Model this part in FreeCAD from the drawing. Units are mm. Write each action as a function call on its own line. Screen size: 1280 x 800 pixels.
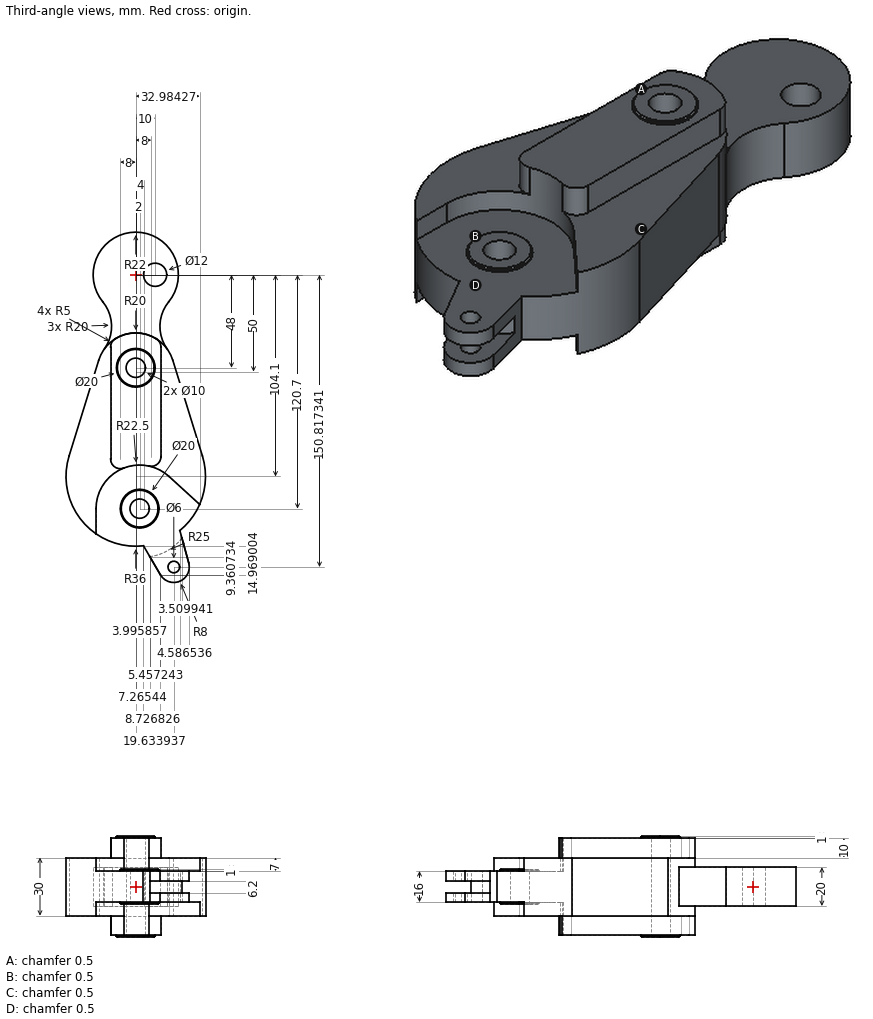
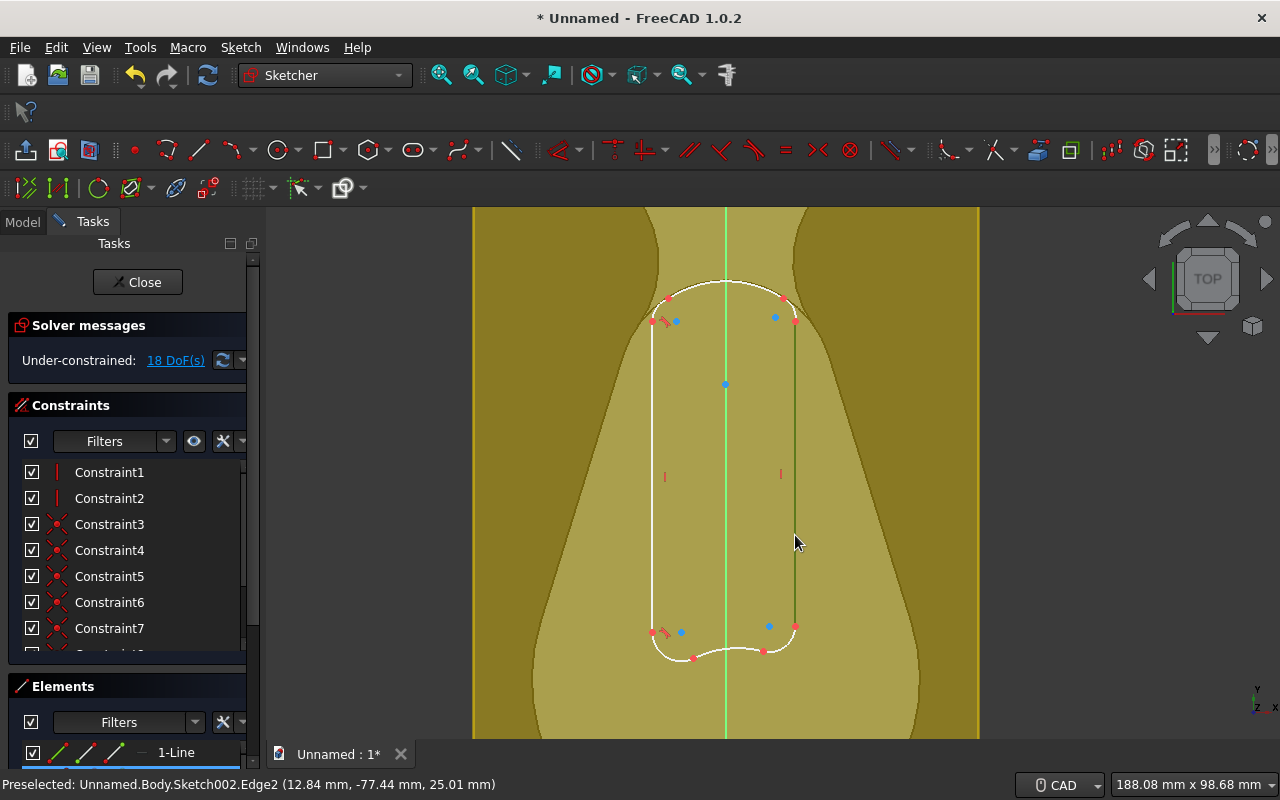
click(777, 651)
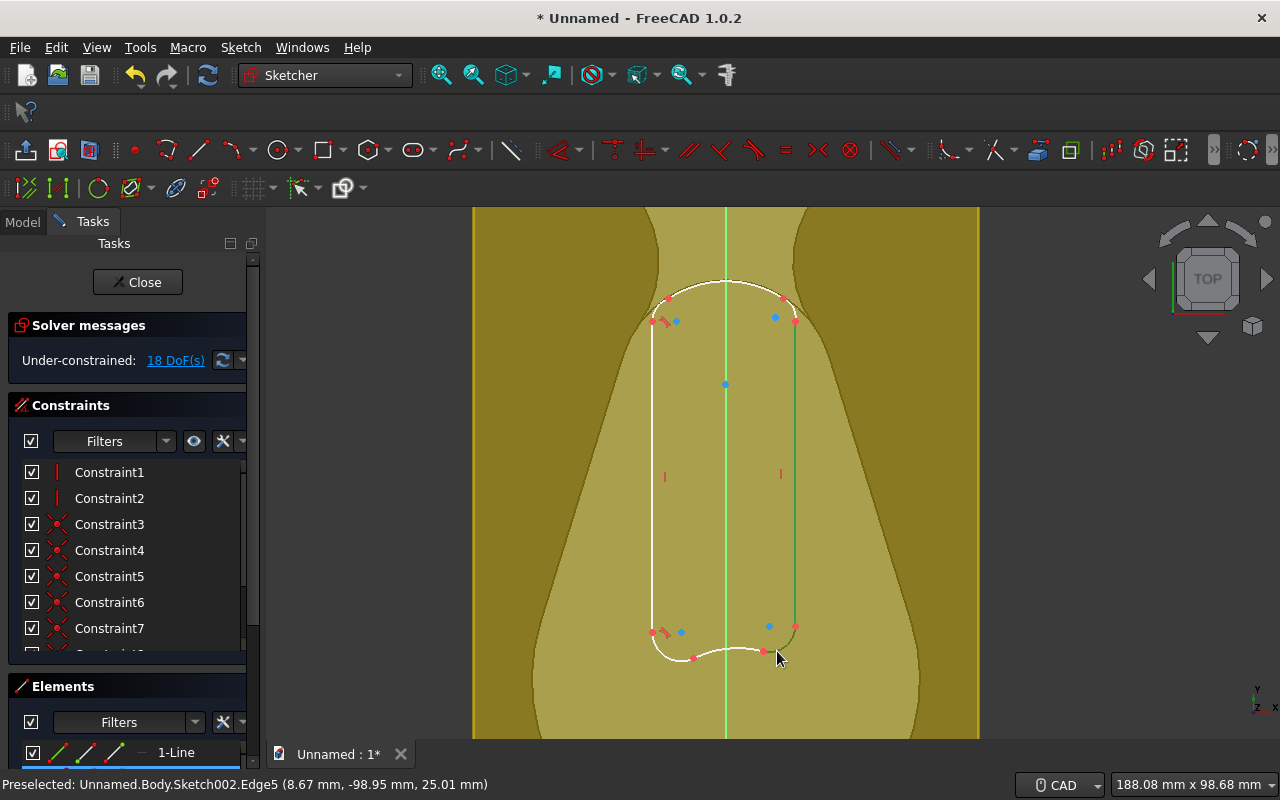
click(754, 150)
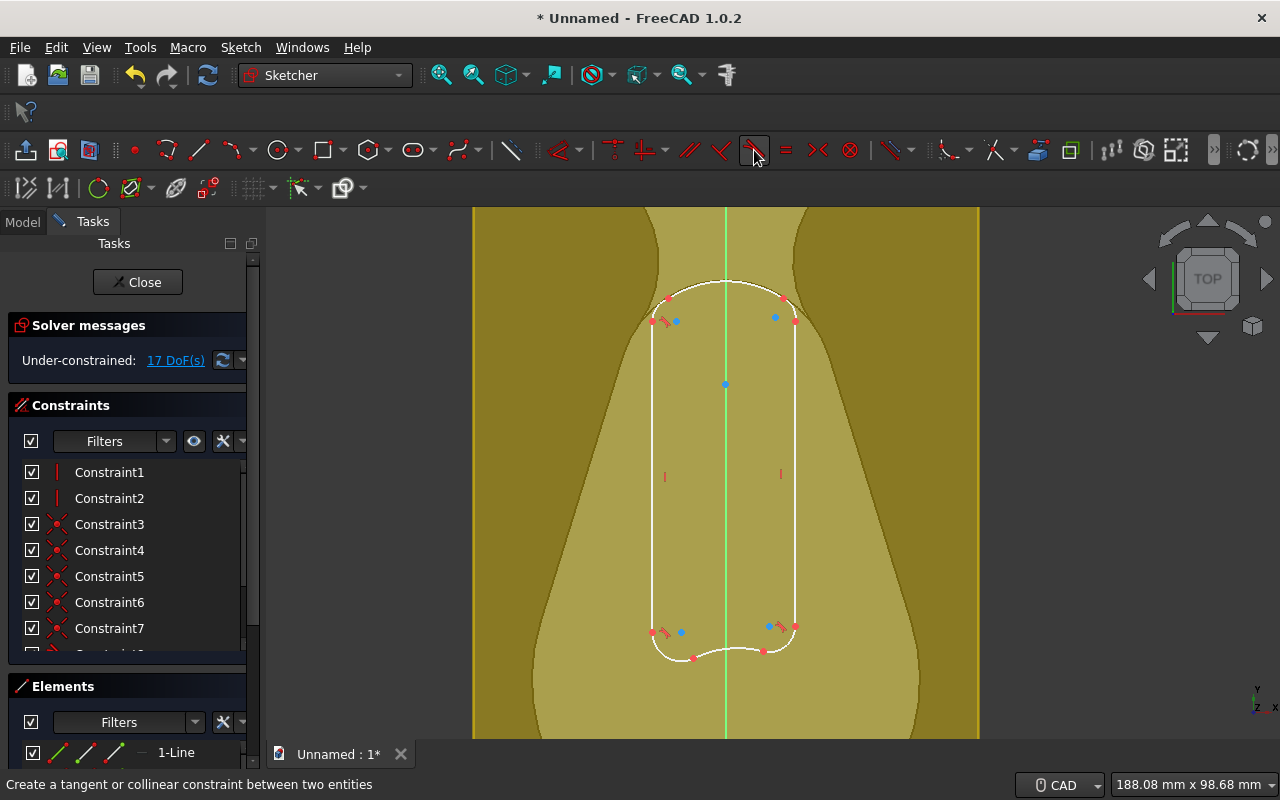
click(795, 535)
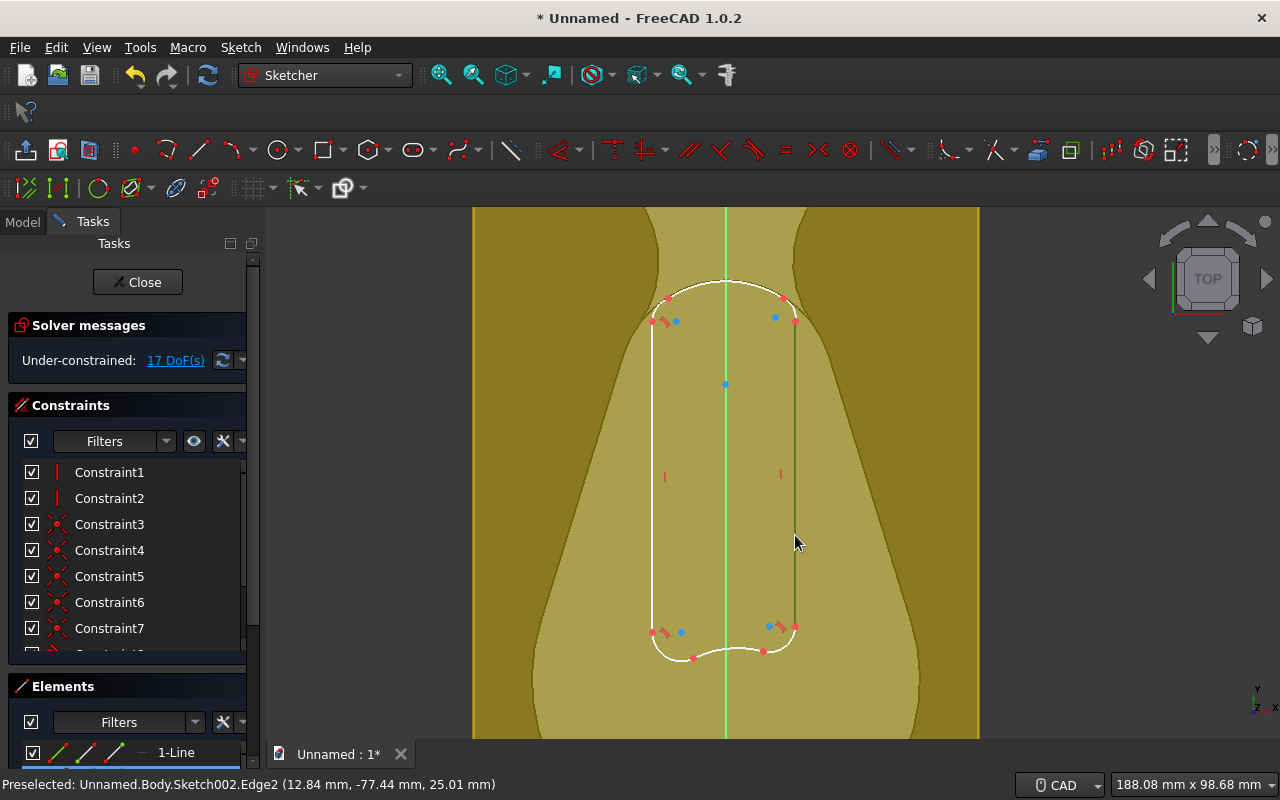
click(793, 308)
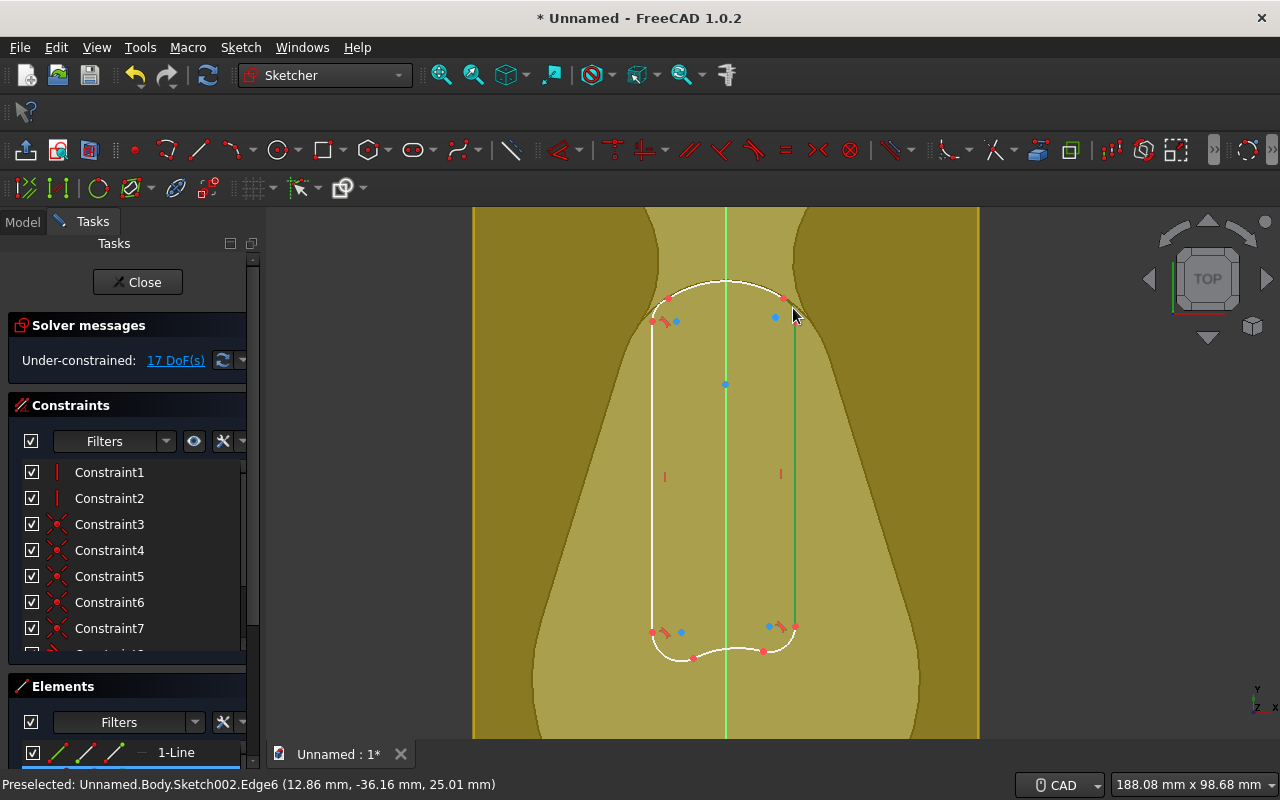
click(754, 150)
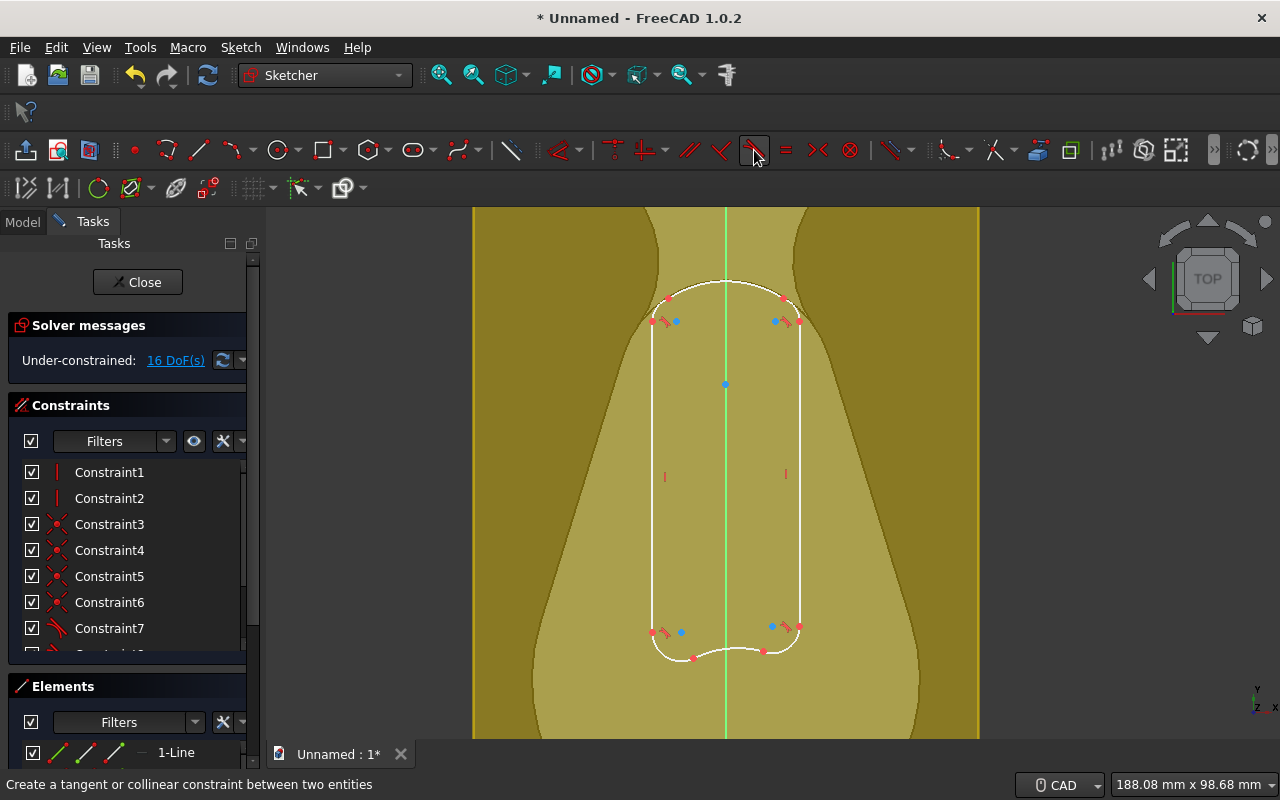
click(657, 648)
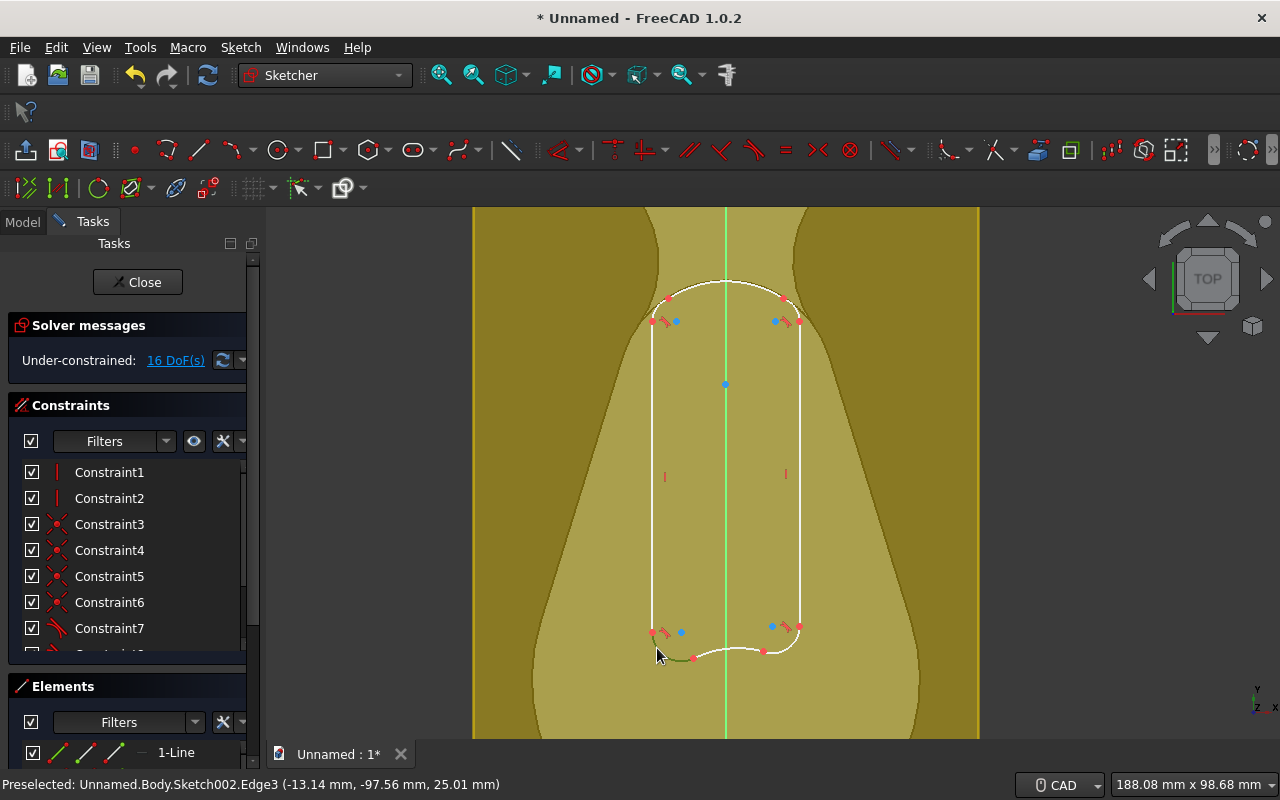
click(742, 648)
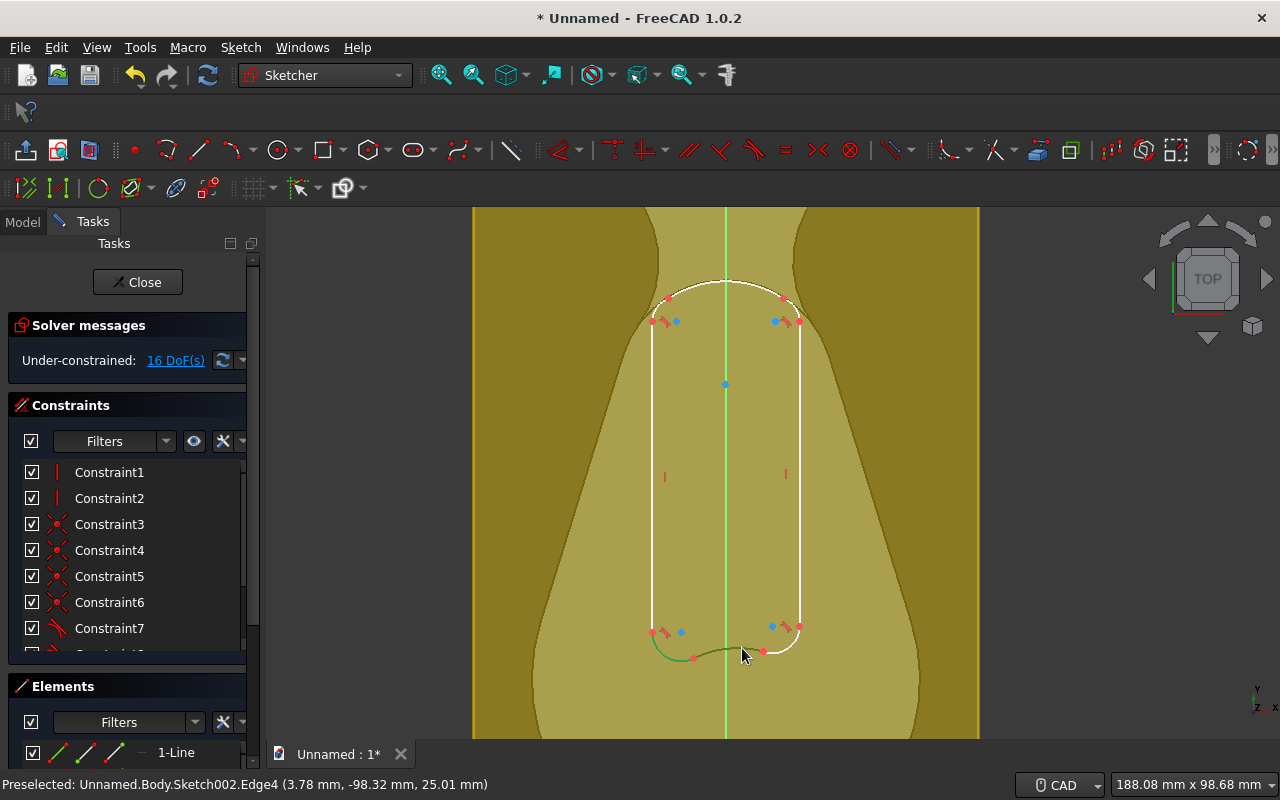
click(754, 150)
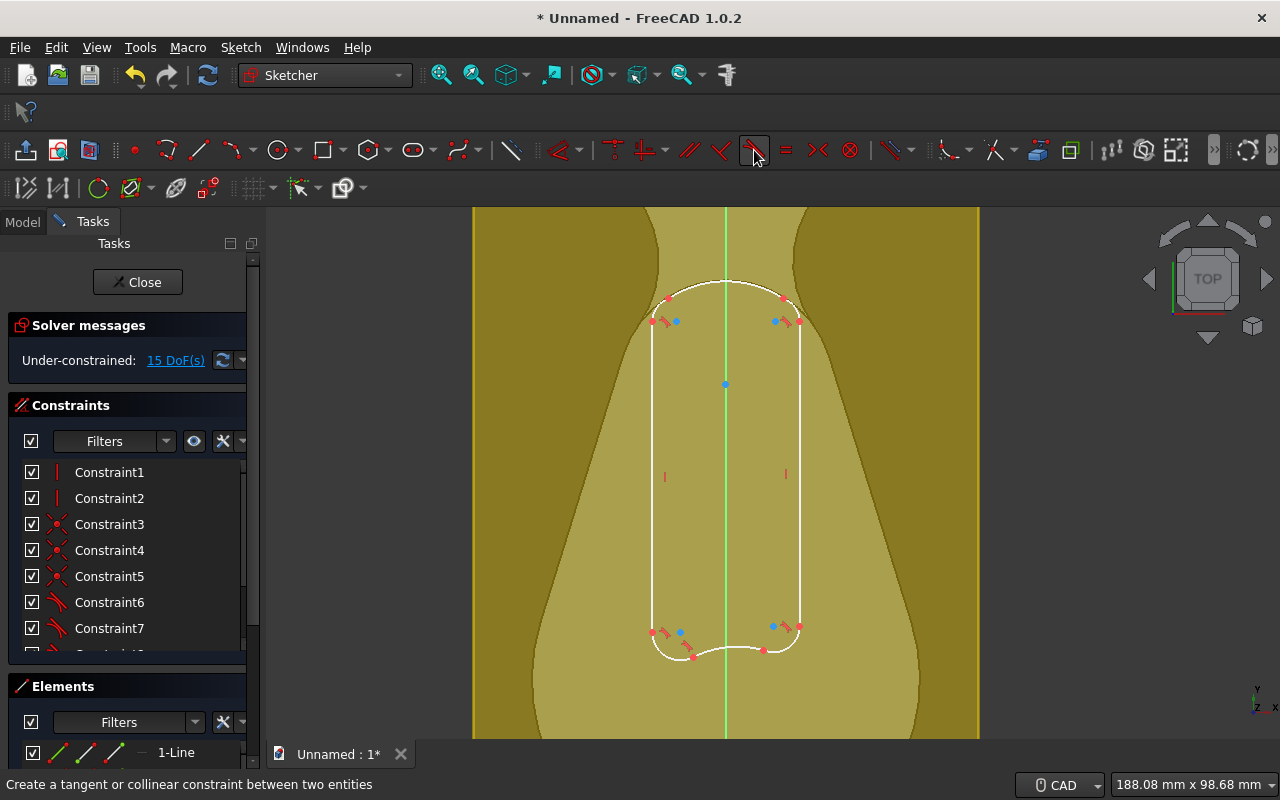
click(742, 647)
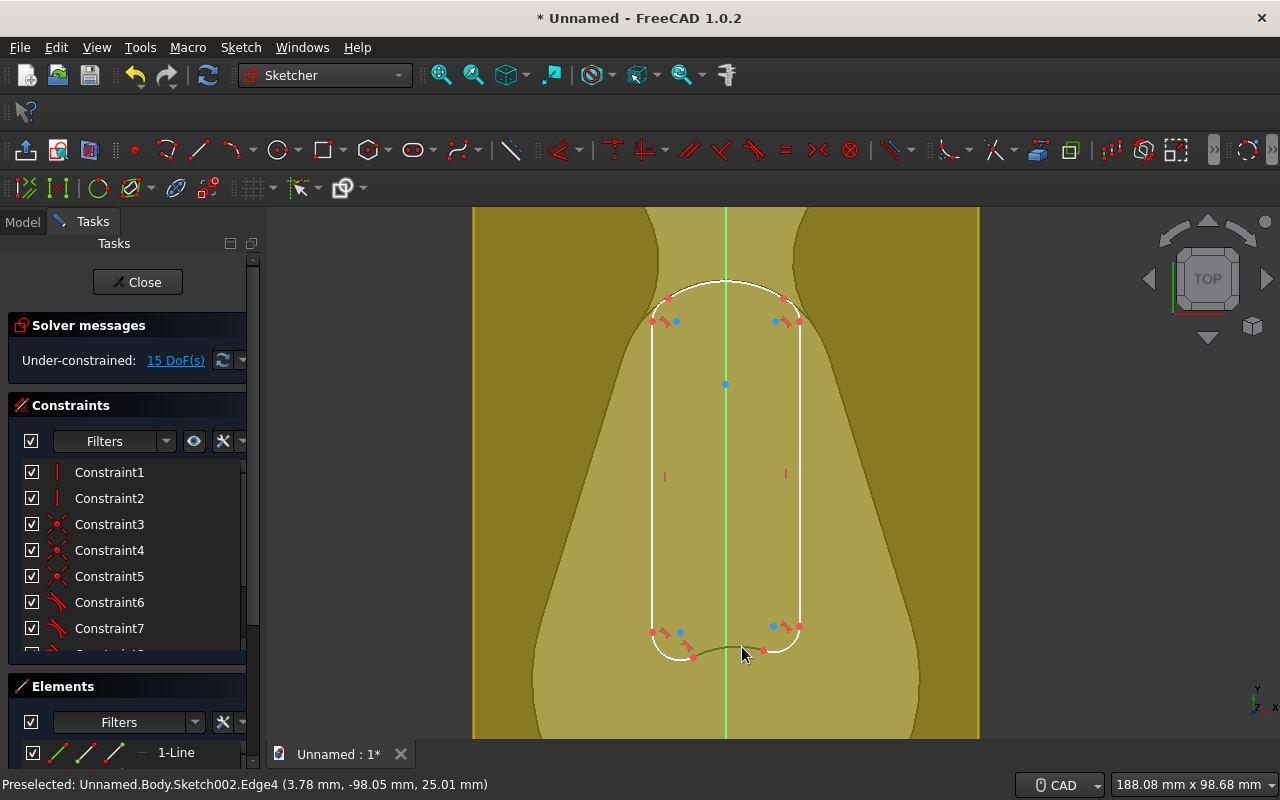
click(778, 652)